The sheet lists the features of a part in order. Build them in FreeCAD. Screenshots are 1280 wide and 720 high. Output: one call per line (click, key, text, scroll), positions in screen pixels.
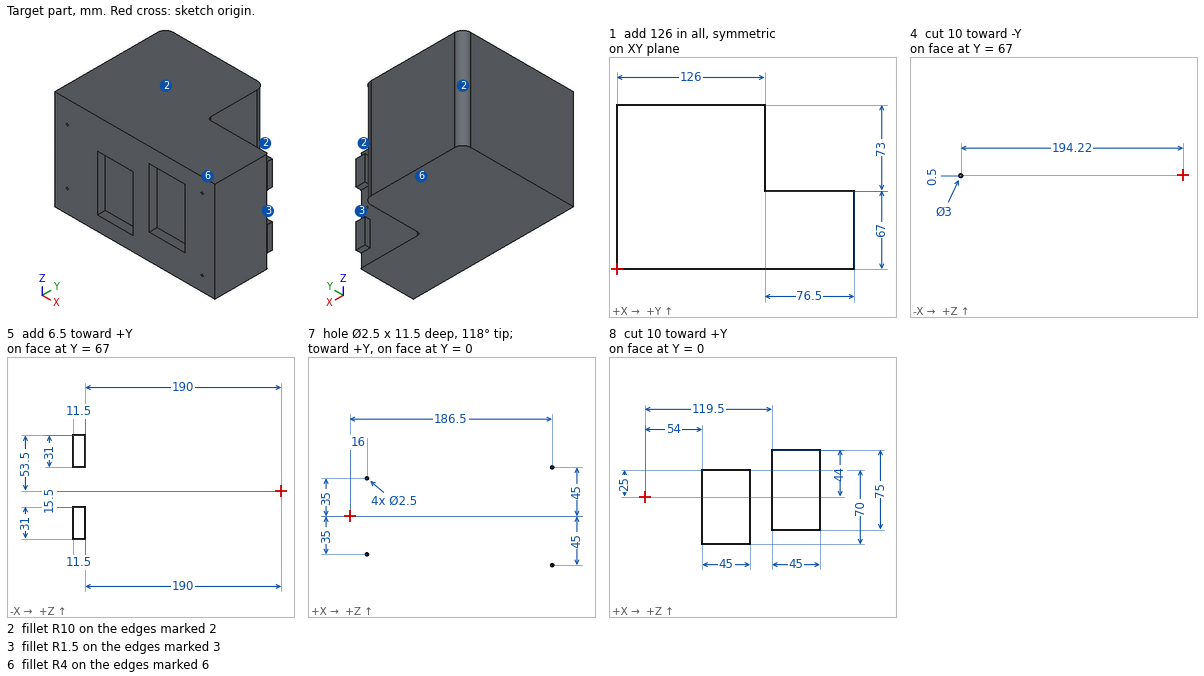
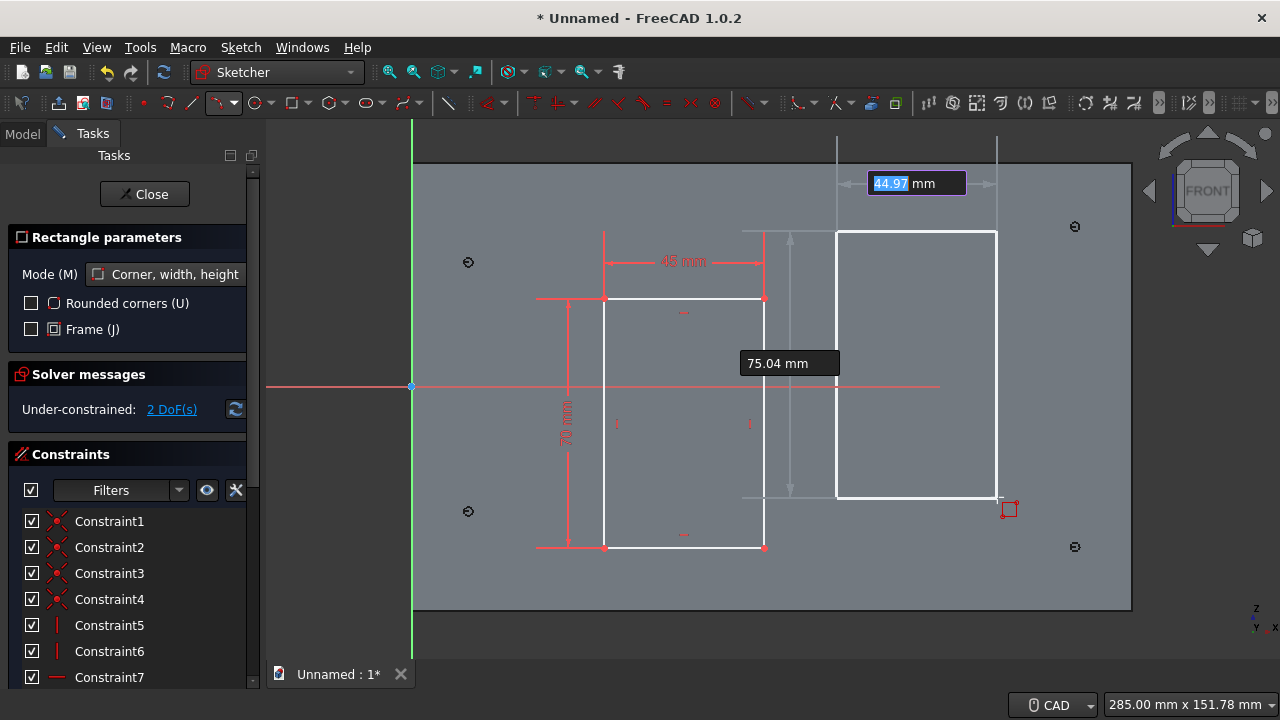
text(45)
key(Tab)
text(75)
key(Return)
key(Escape)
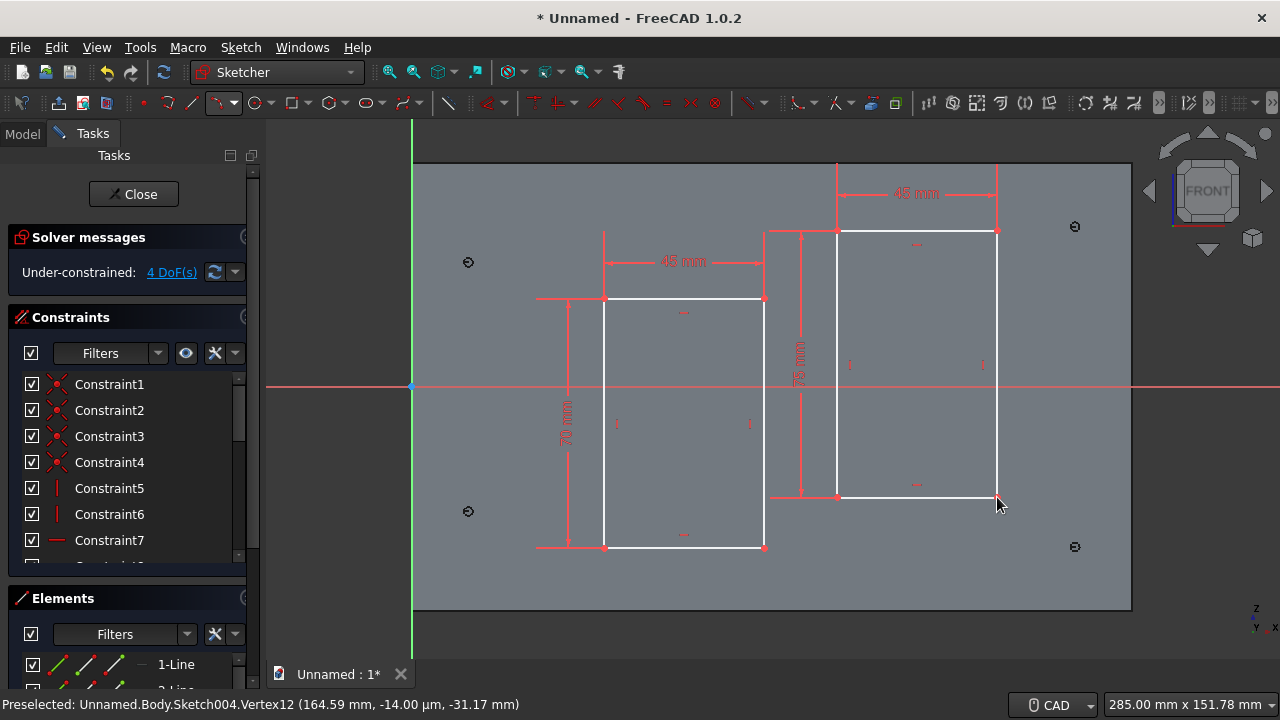
key(d)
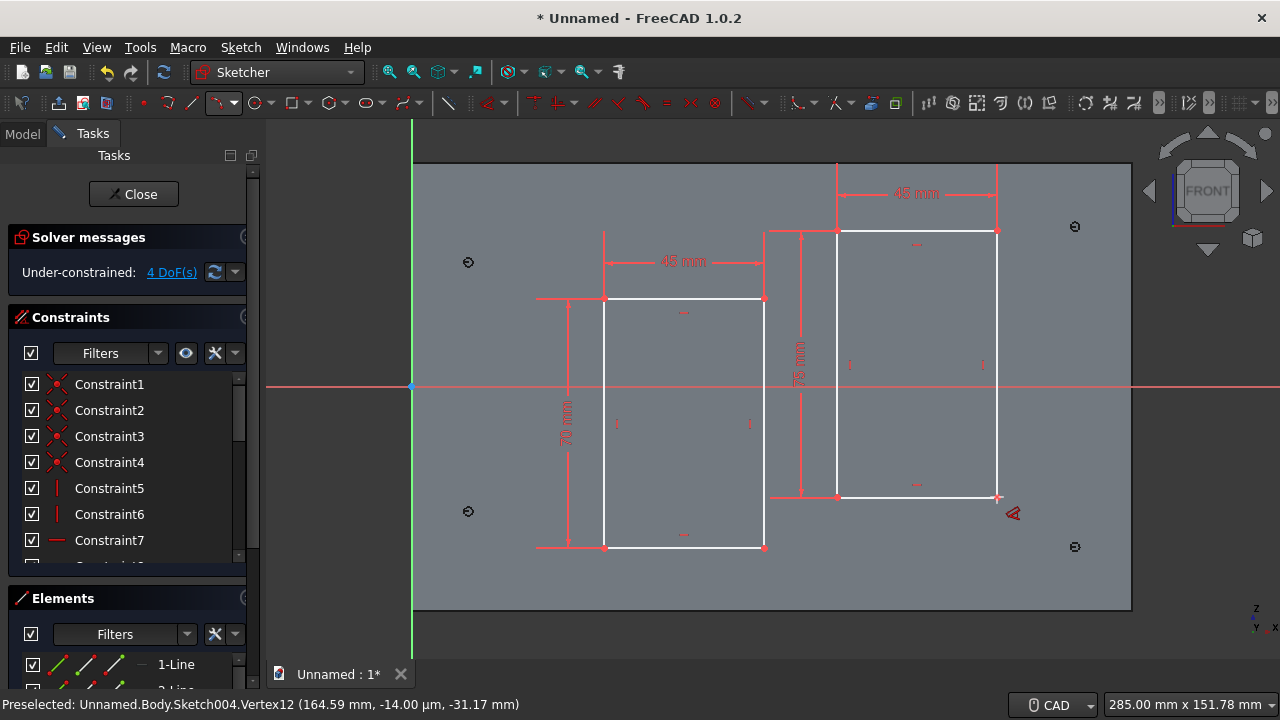
click(604, 299)
click(508, 265)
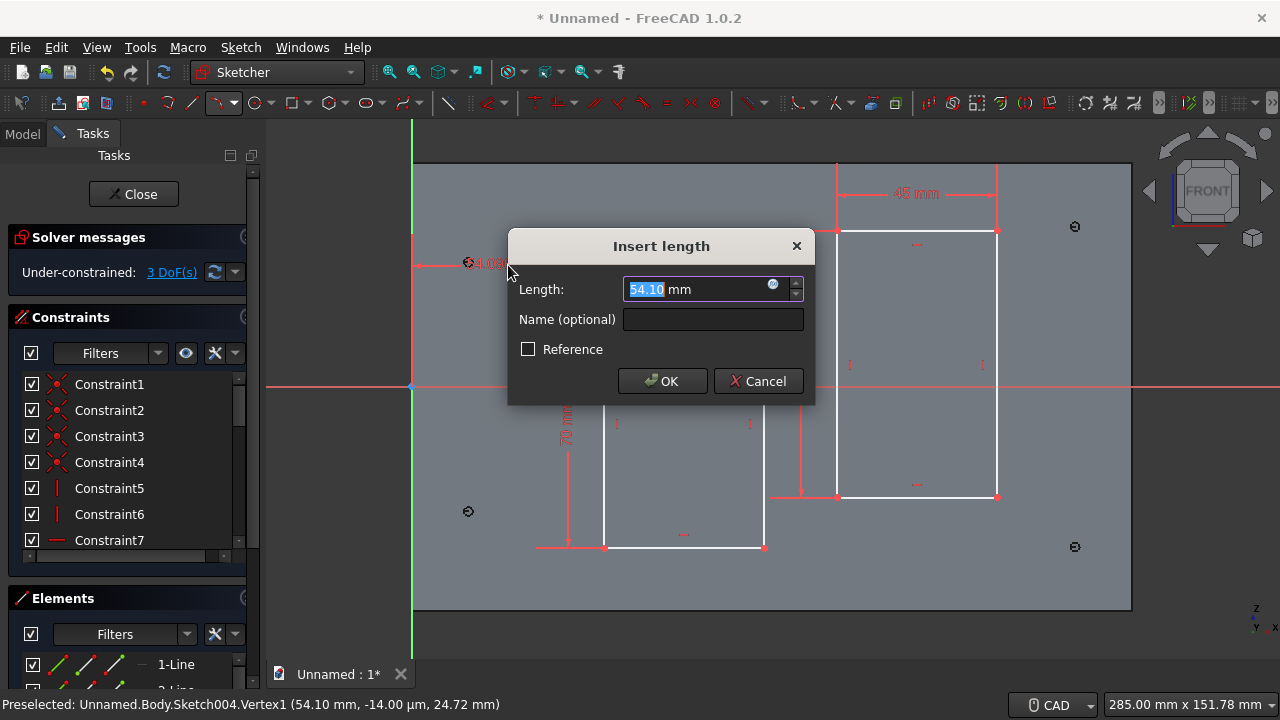
text(54)
key(Return)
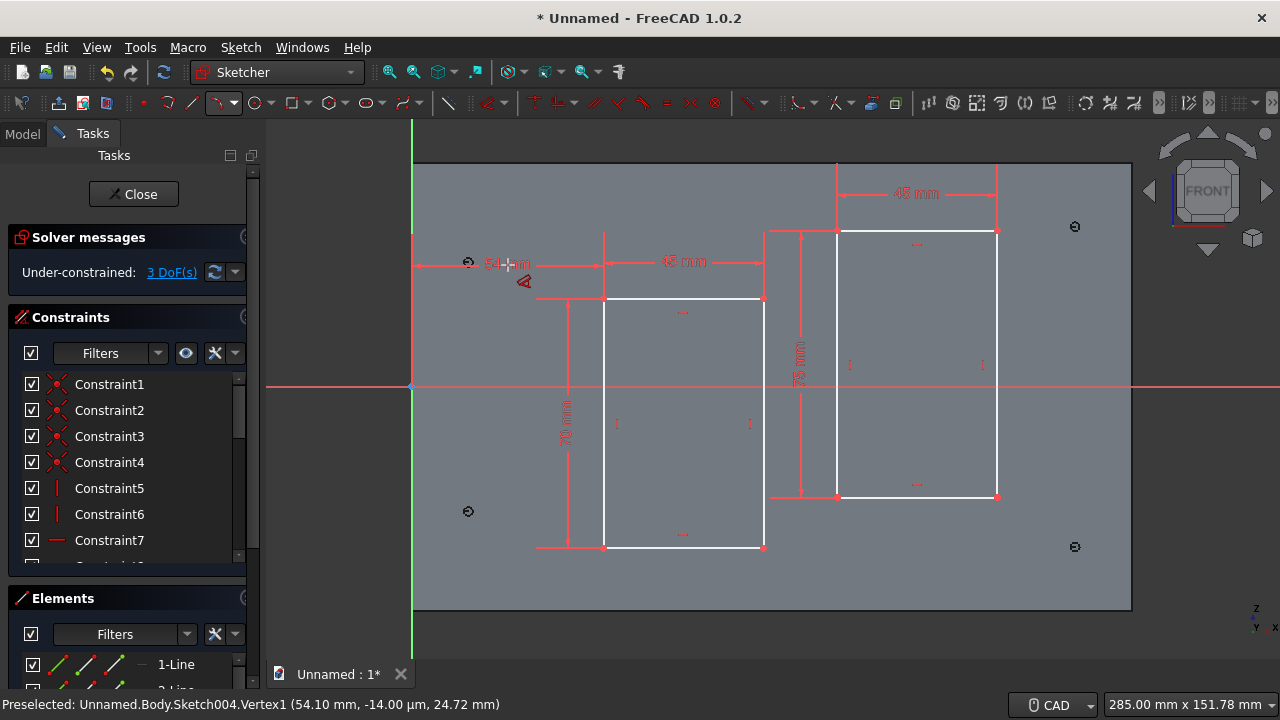
click(604, 299)
click(378, 343)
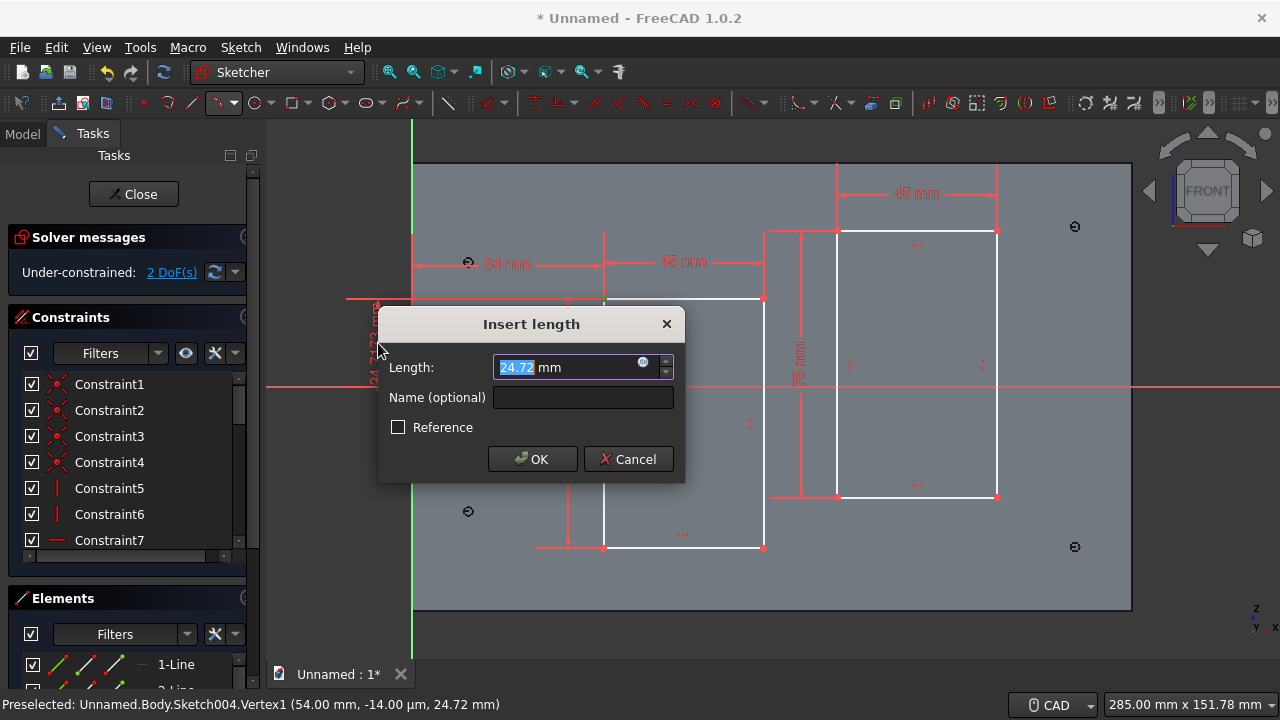
text(25)
key(Return)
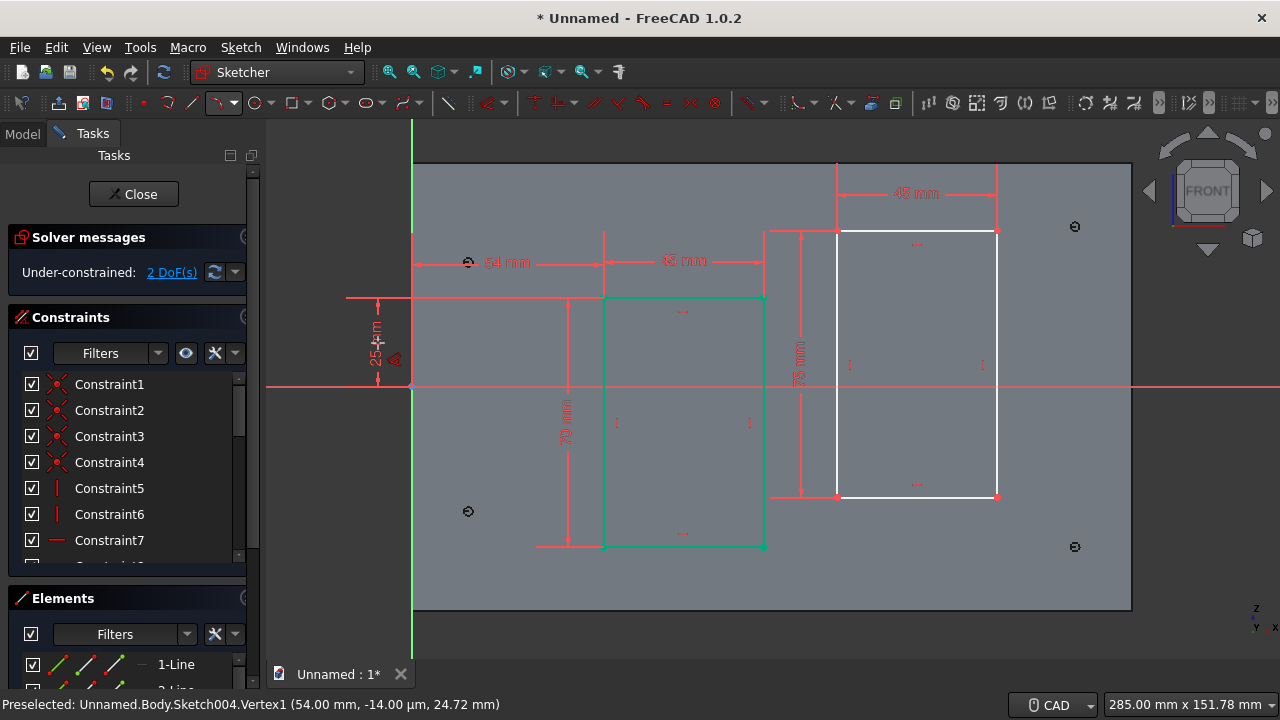
click(837, 231)
click(378, 309)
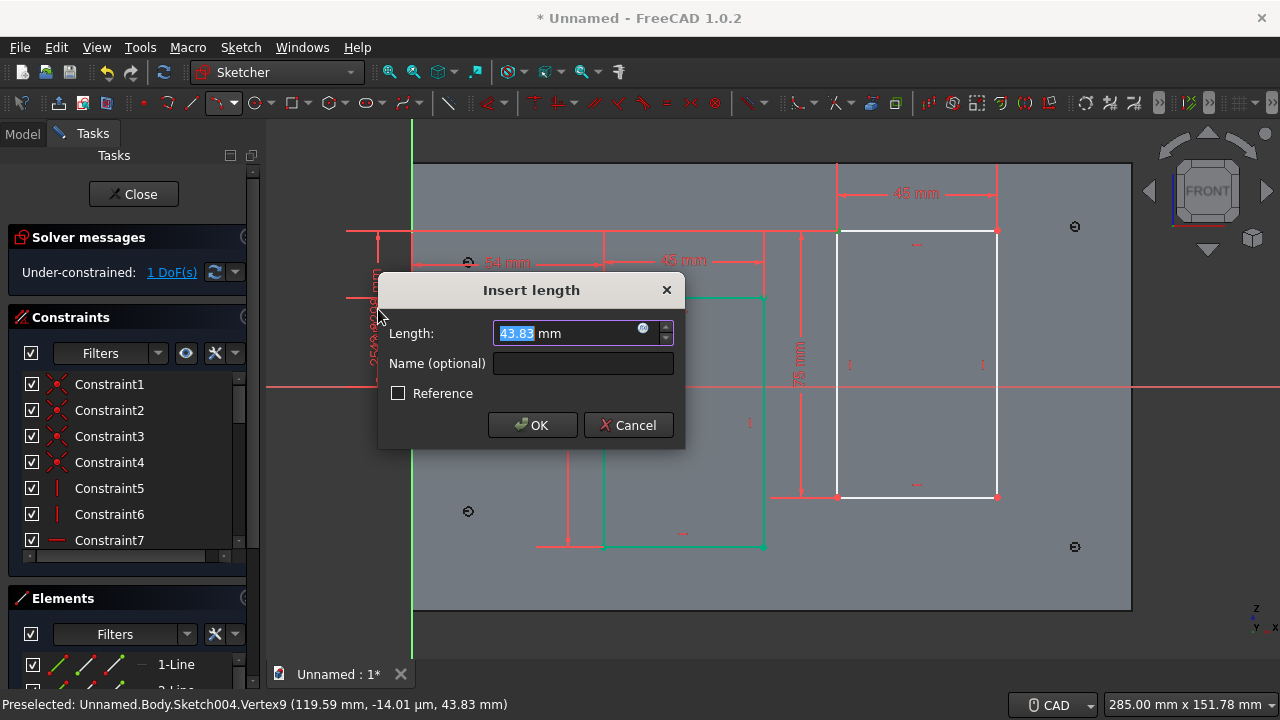
text(44)
key(Return)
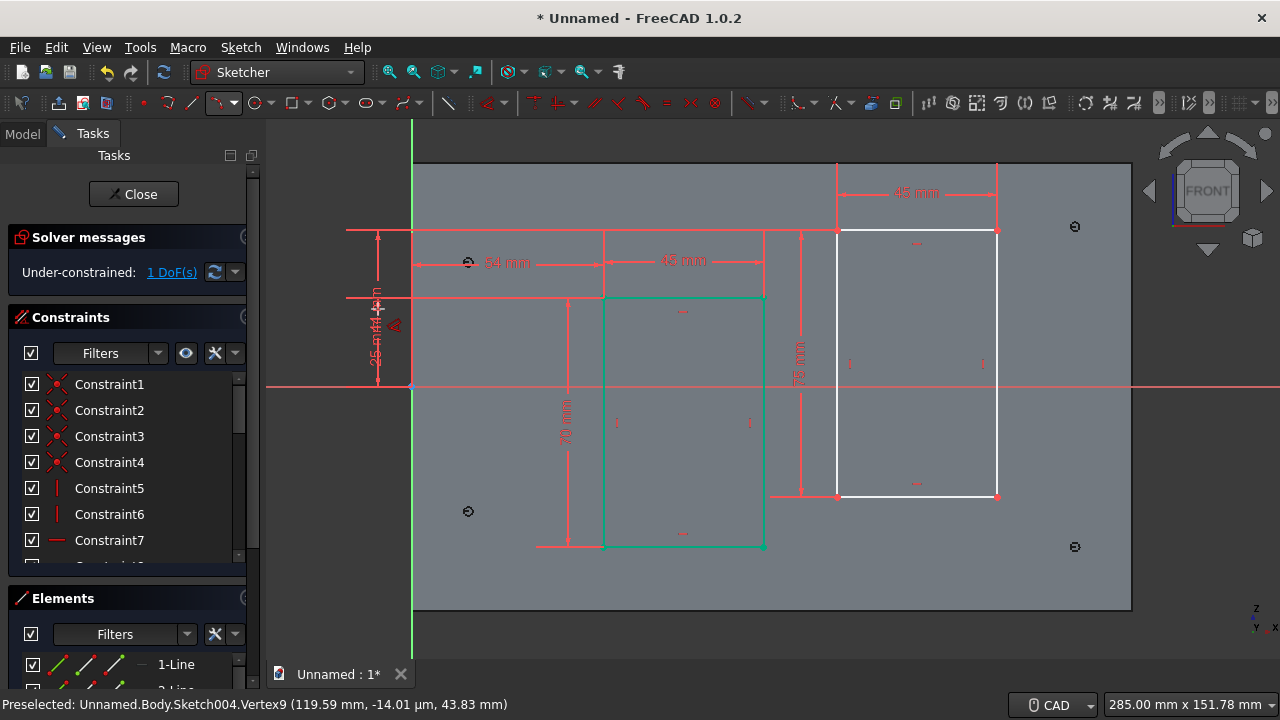
click(837, 230)
click(624, 196)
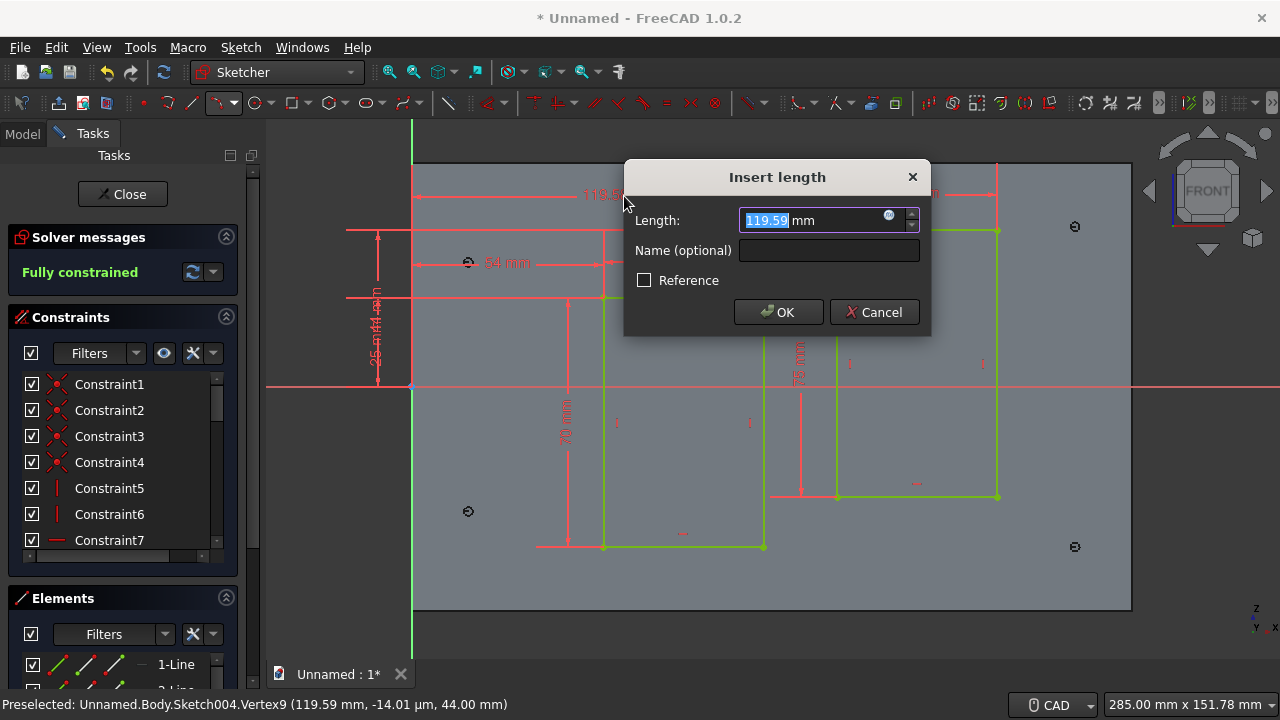
text(119.5)
key(Return)
key(Escape)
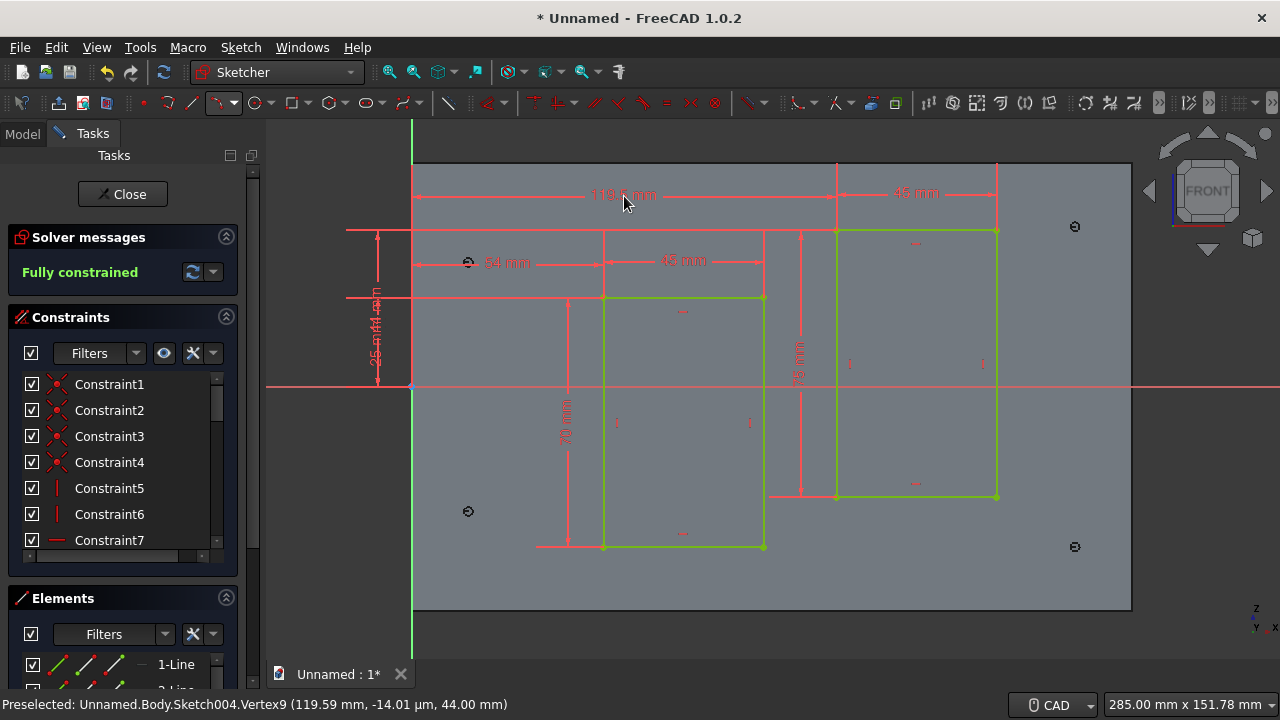
click(123, 194)